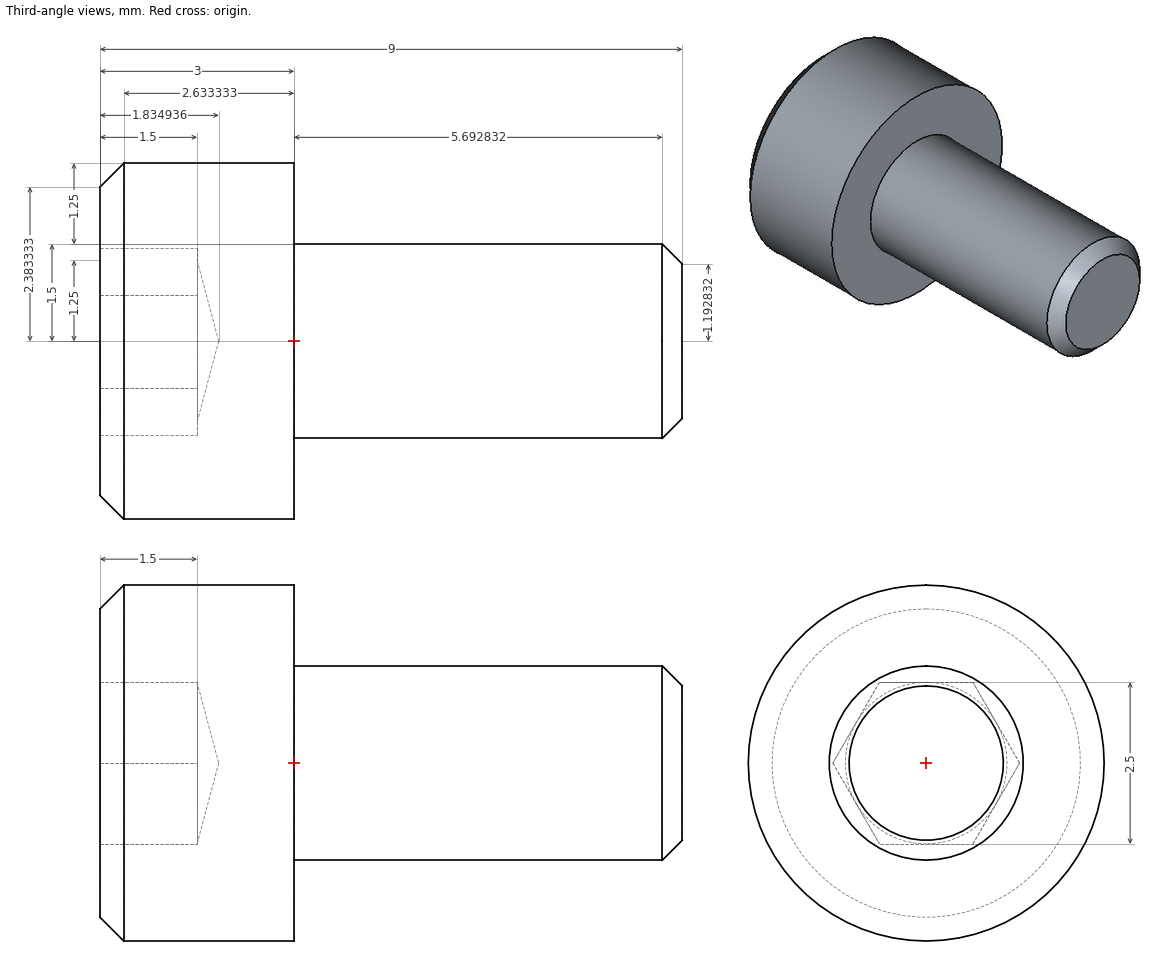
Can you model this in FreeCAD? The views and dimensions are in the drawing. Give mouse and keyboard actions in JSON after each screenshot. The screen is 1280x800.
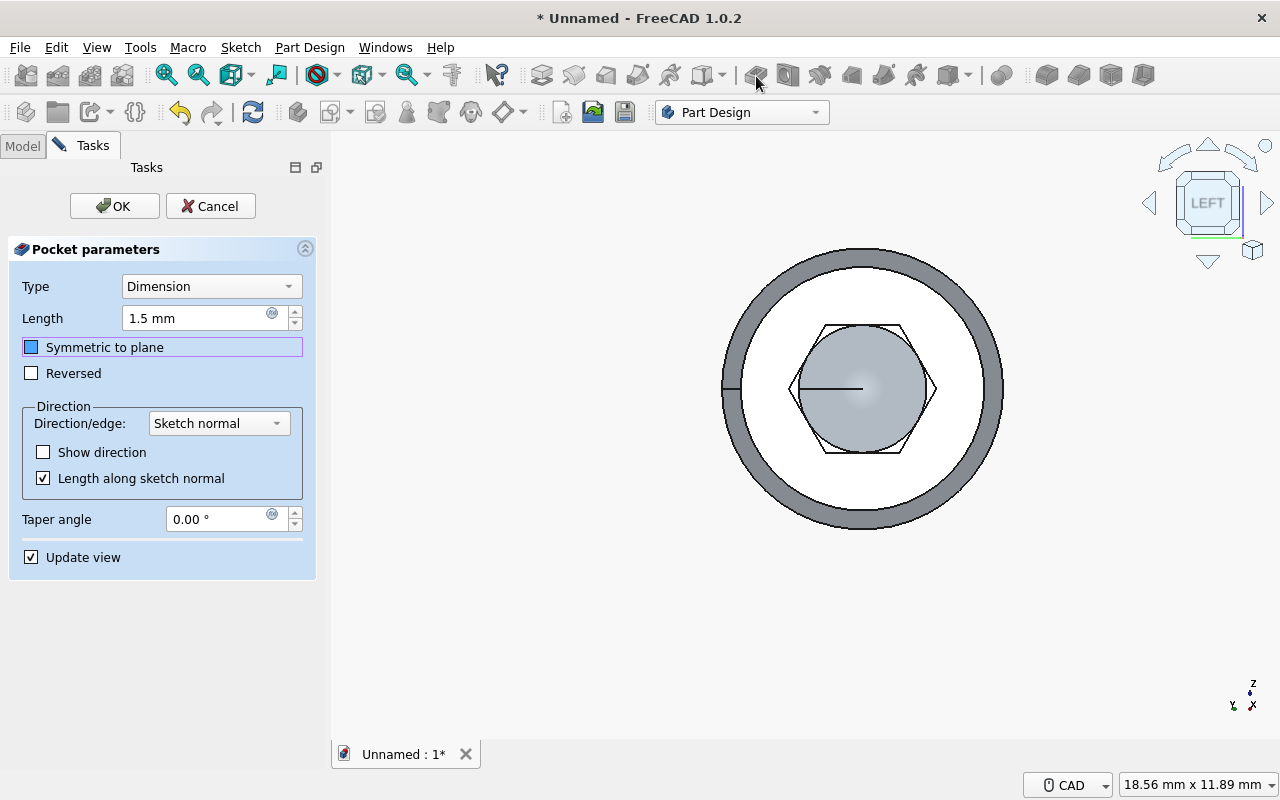
{"action": "left_click", "coordinate": [115, 206]}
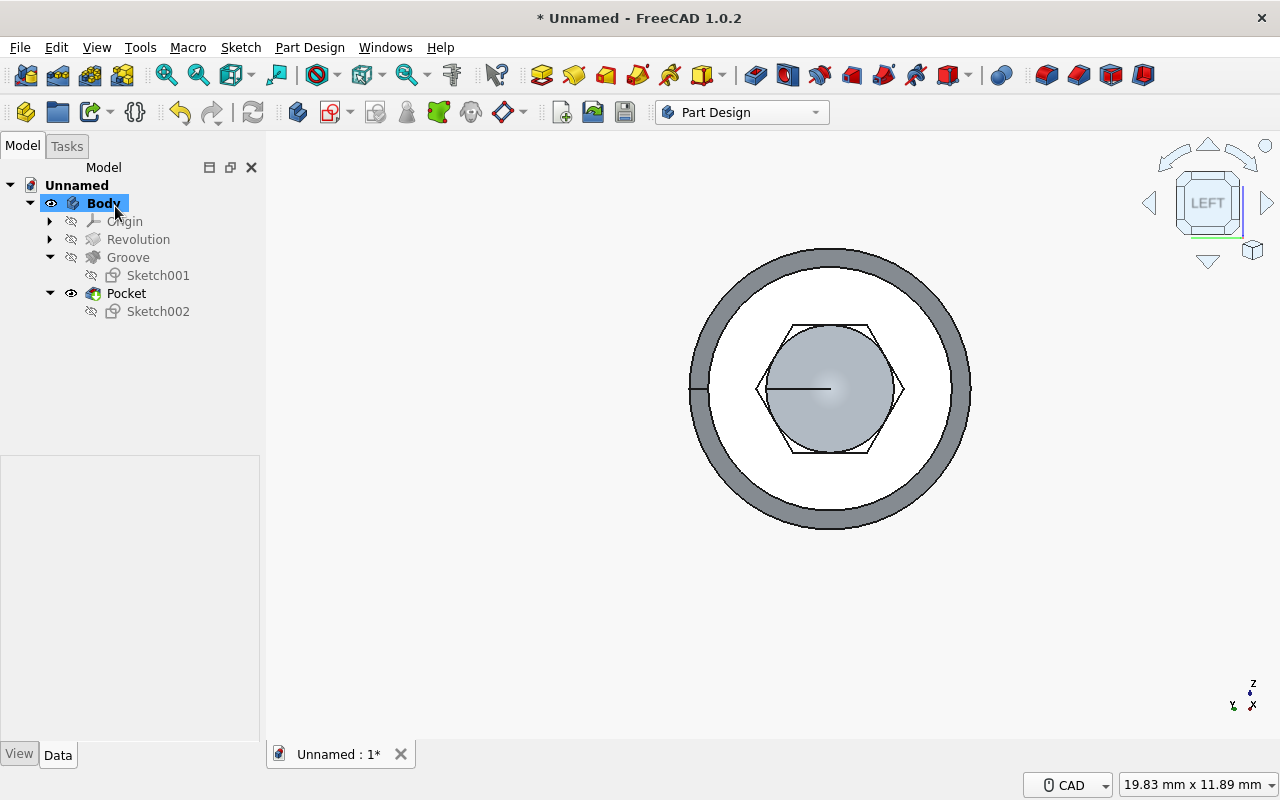
{"action": "key", "text": "0"}